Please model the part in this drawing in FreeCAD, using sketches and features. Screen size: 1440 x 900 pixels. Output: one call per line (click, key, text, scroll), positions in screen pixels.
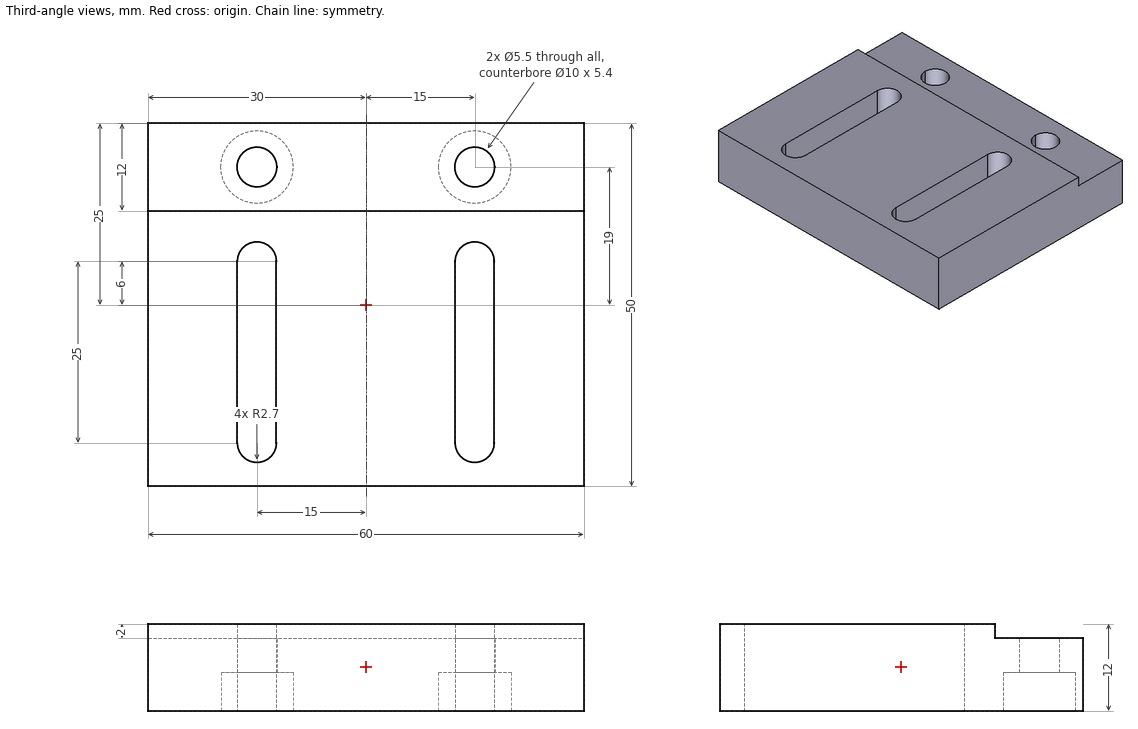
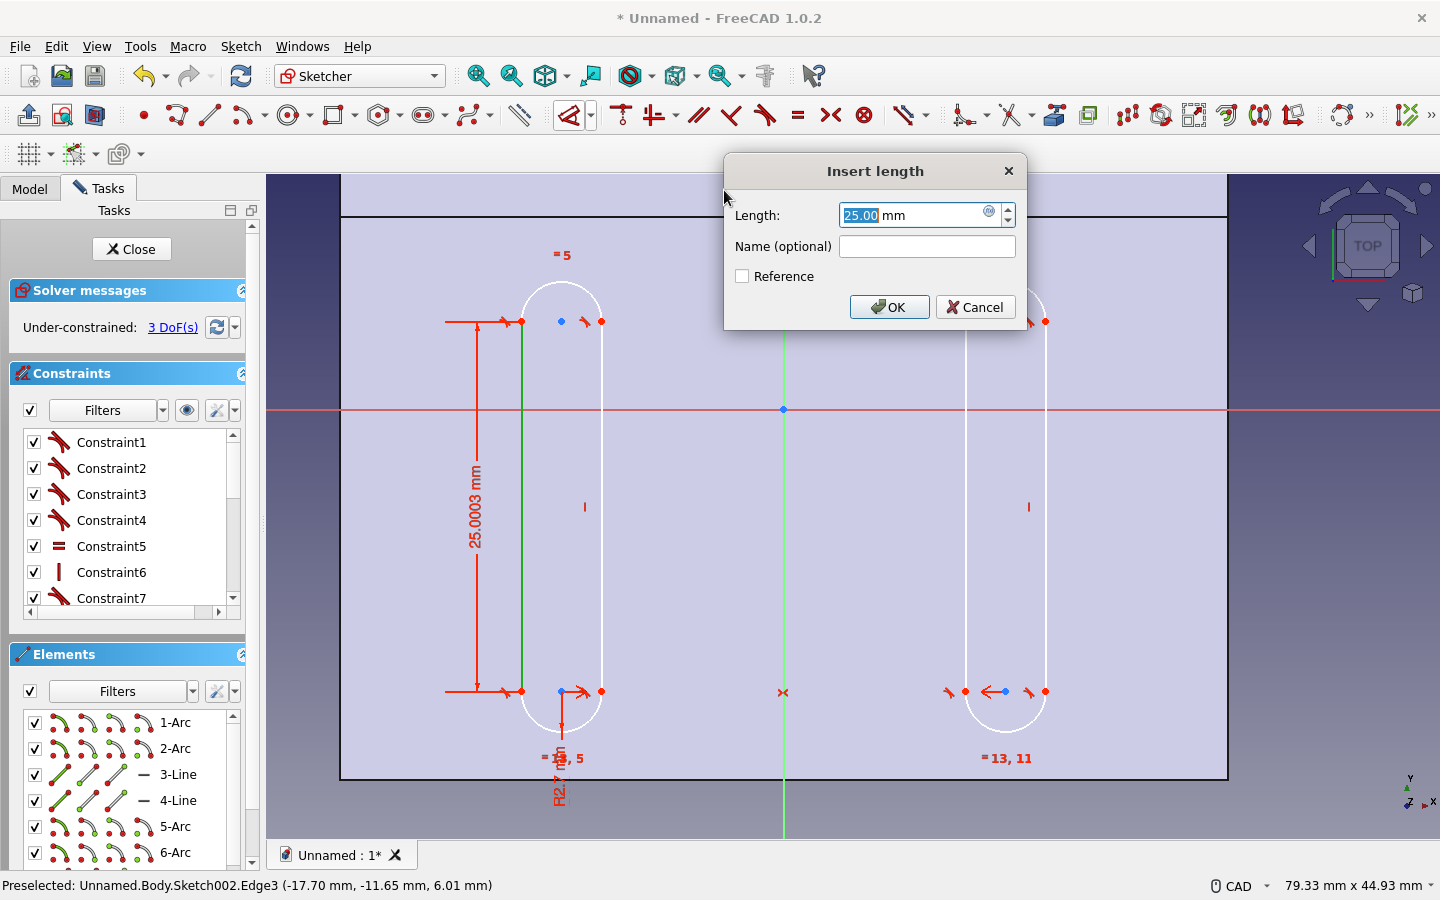
text(25)
key(Return)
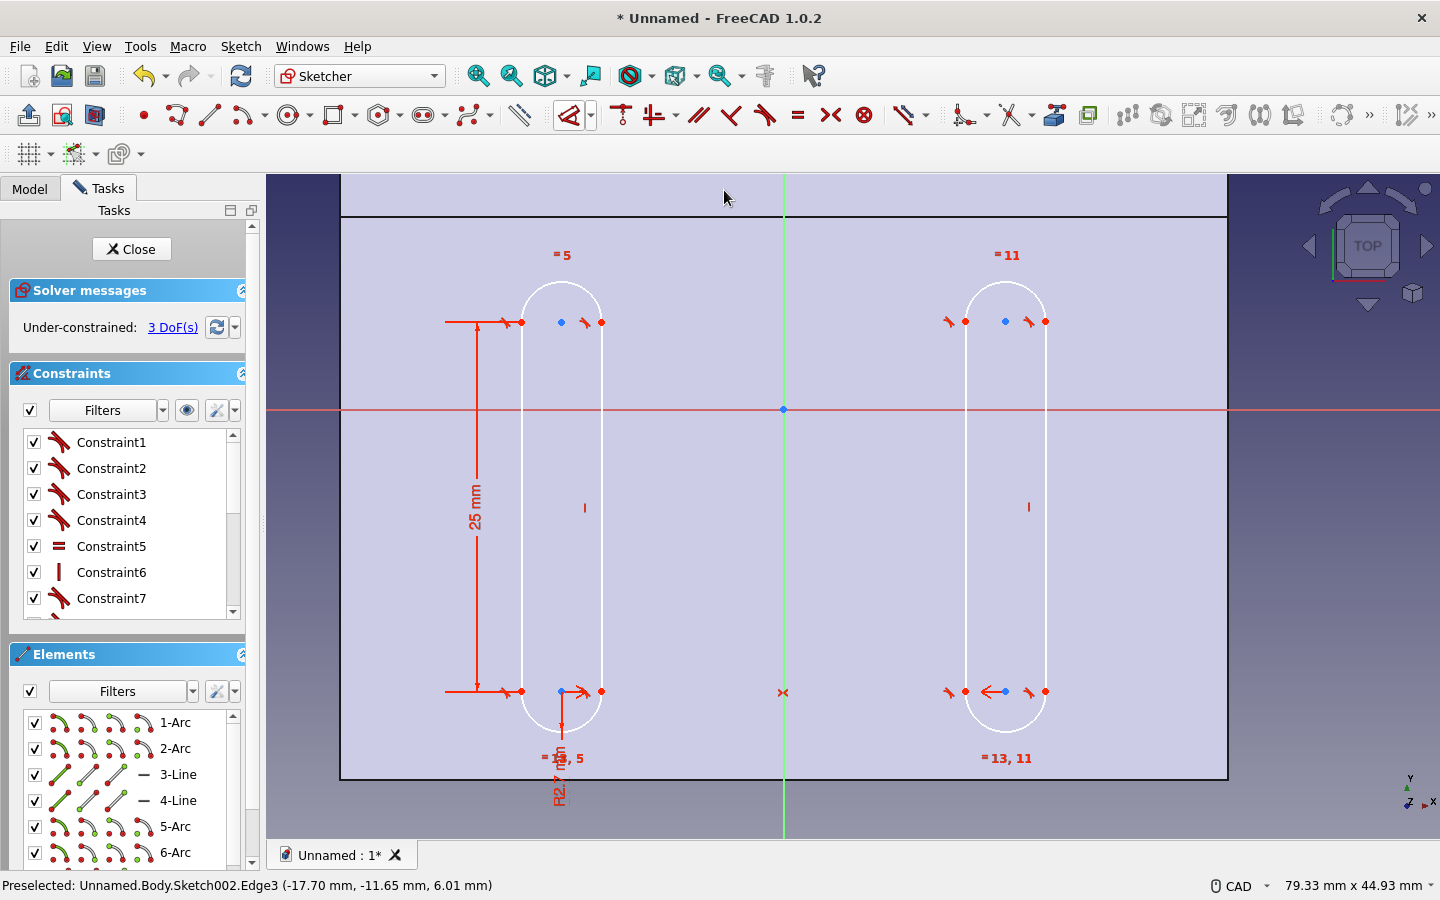
click(966, 581)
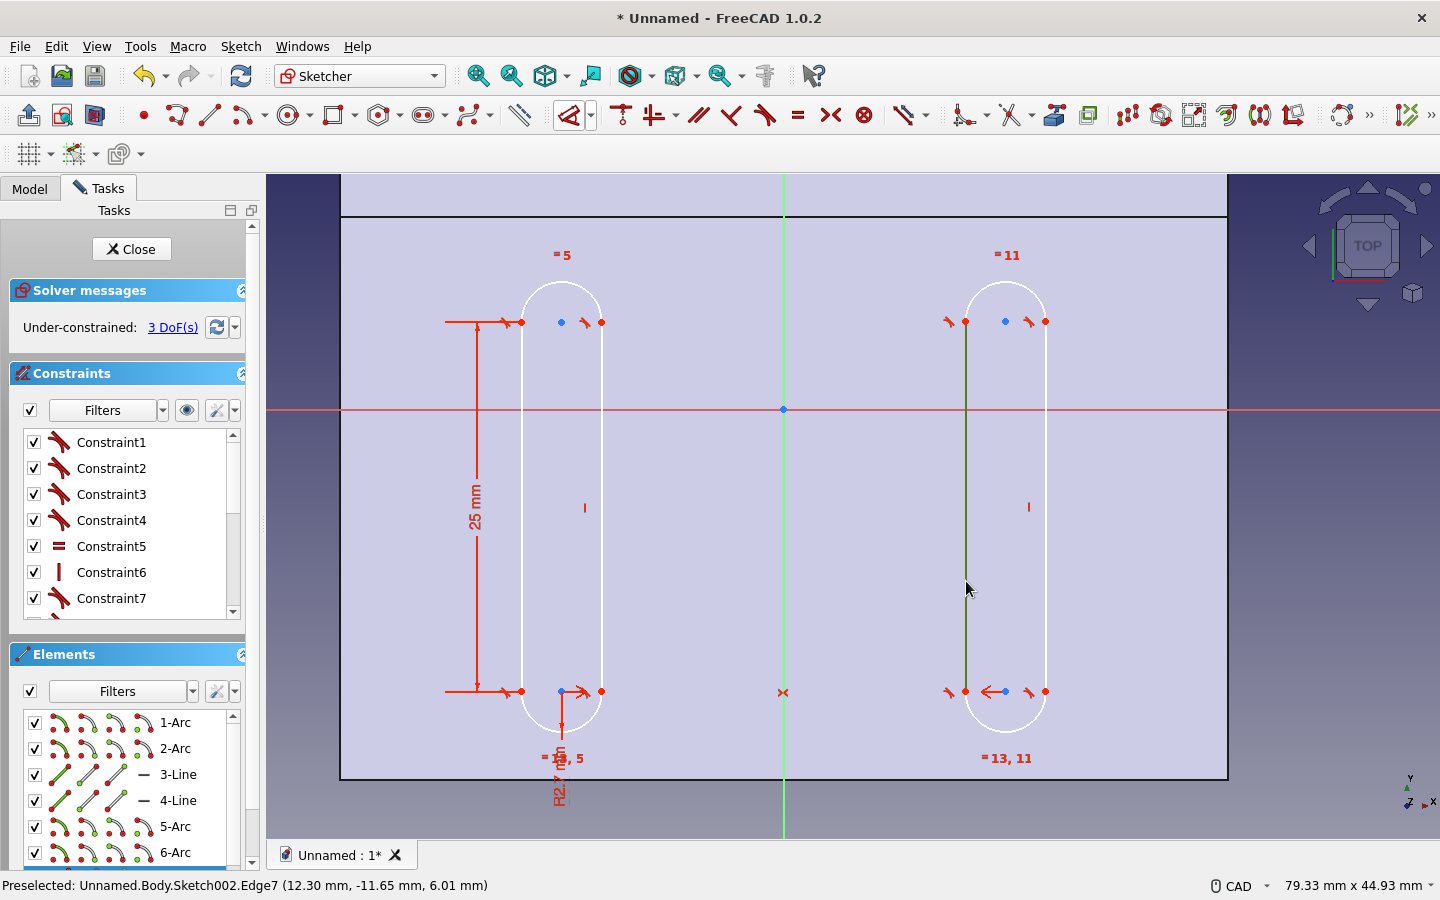
key(i)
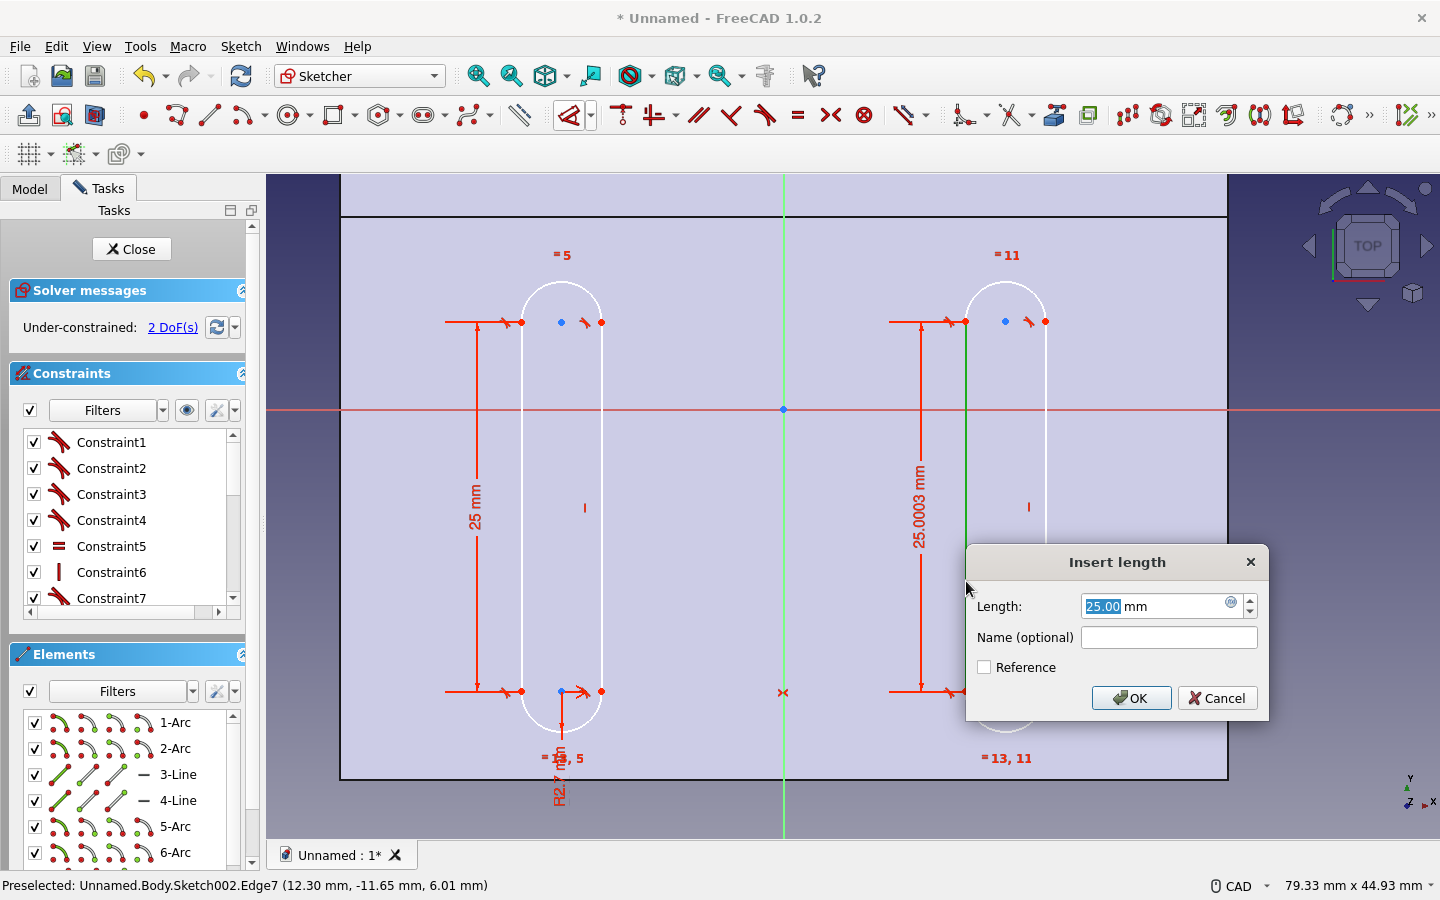
text(25)
key(Return)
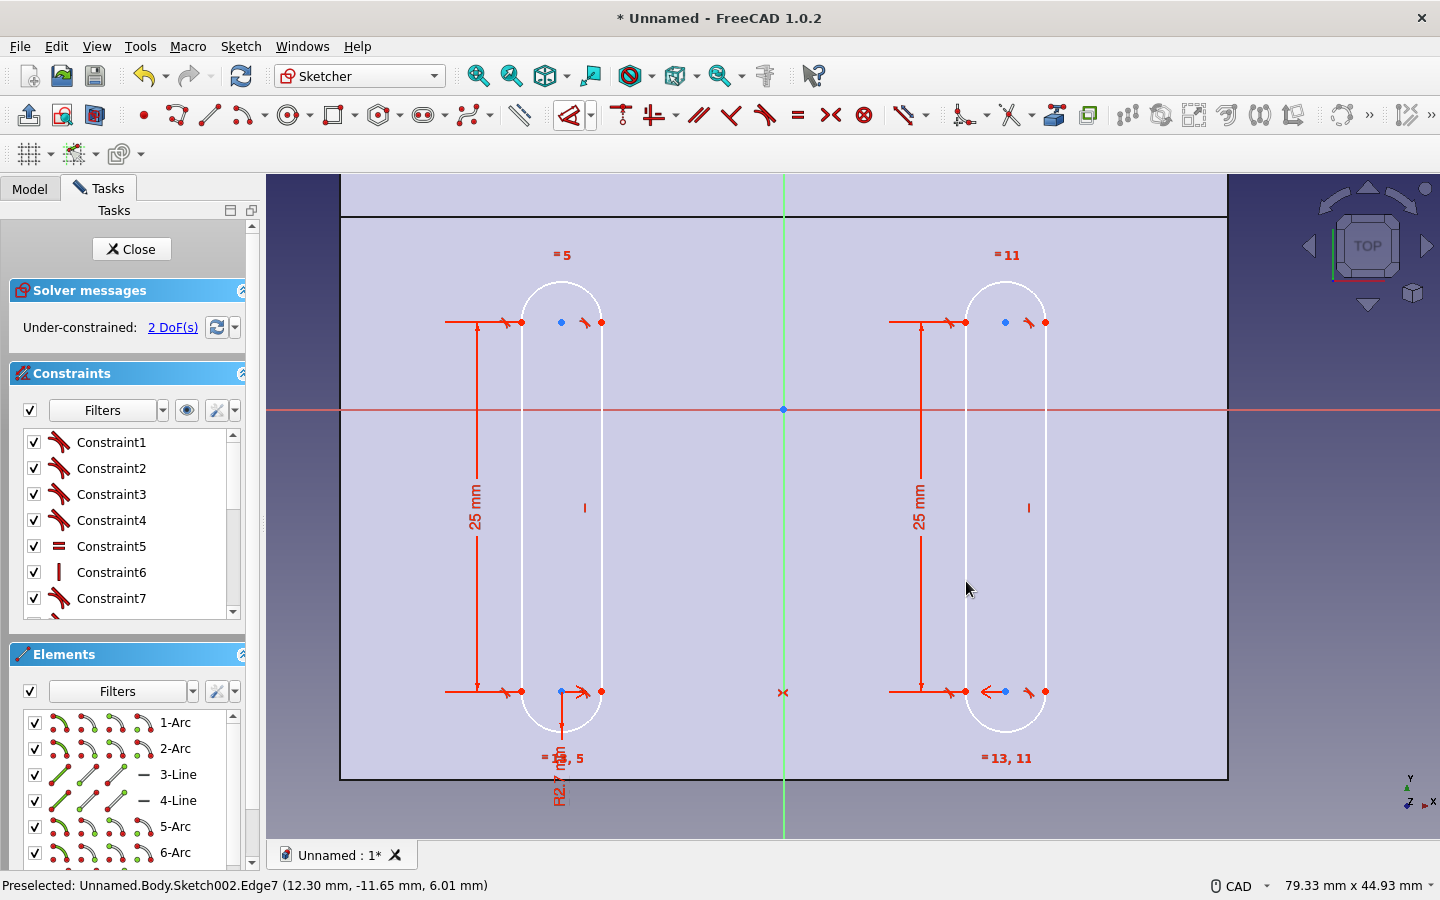
click(602, 322)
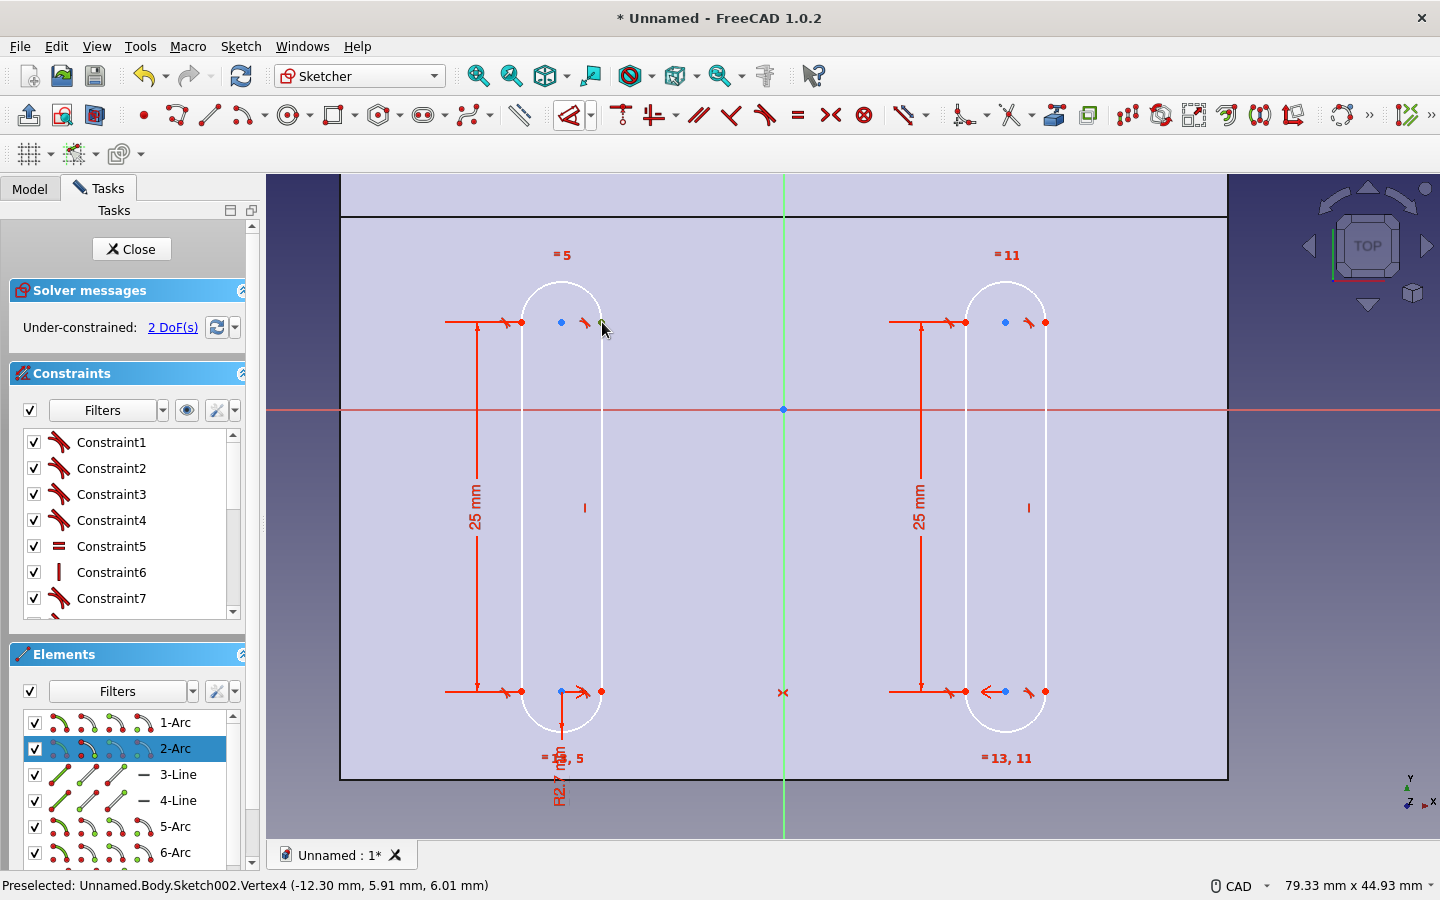
key(i)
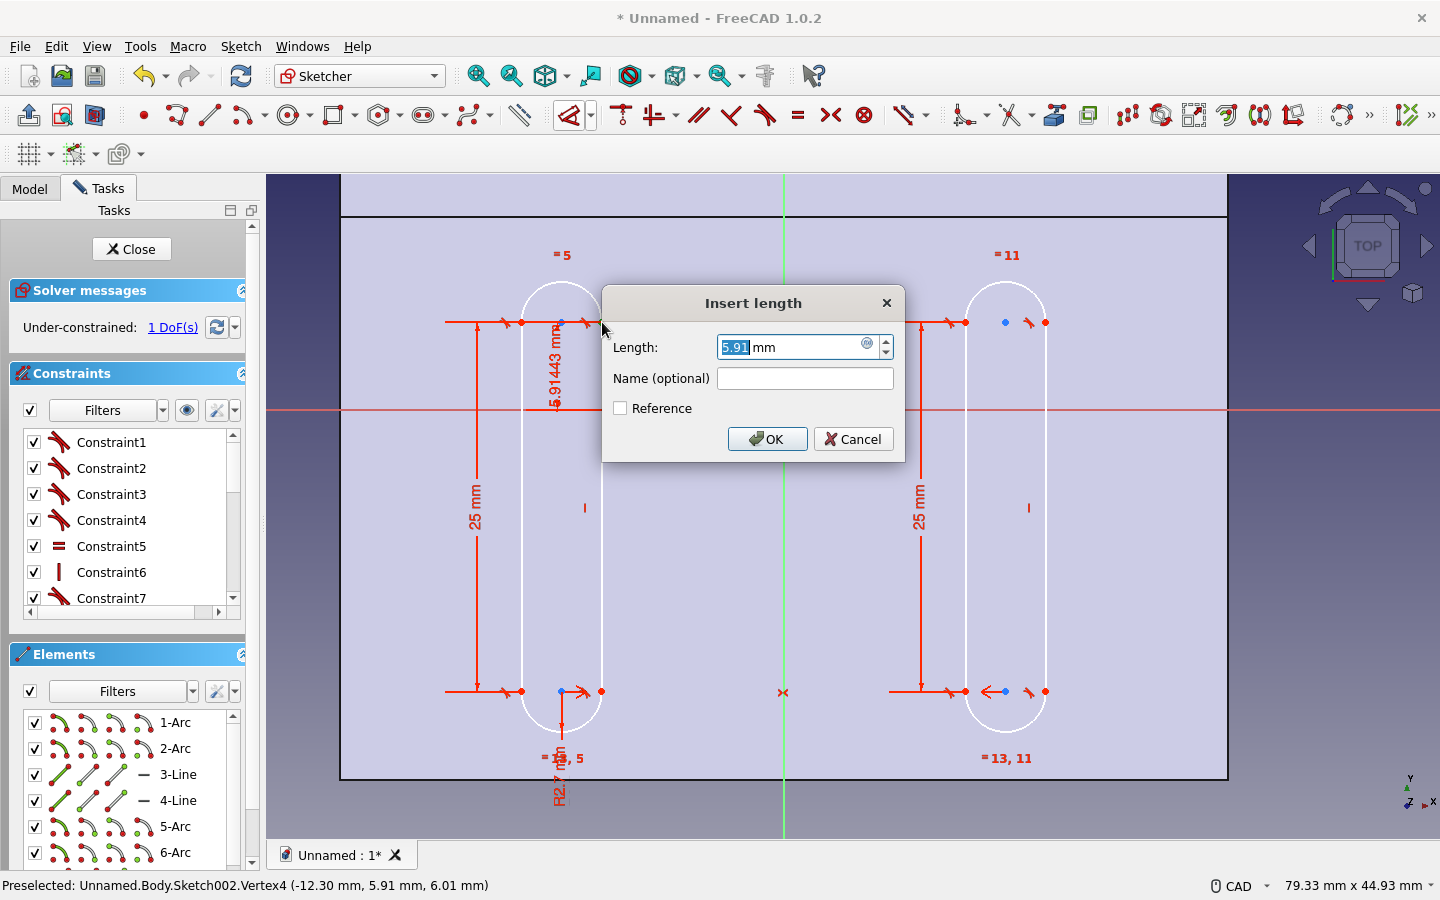
text(6)
key(Return)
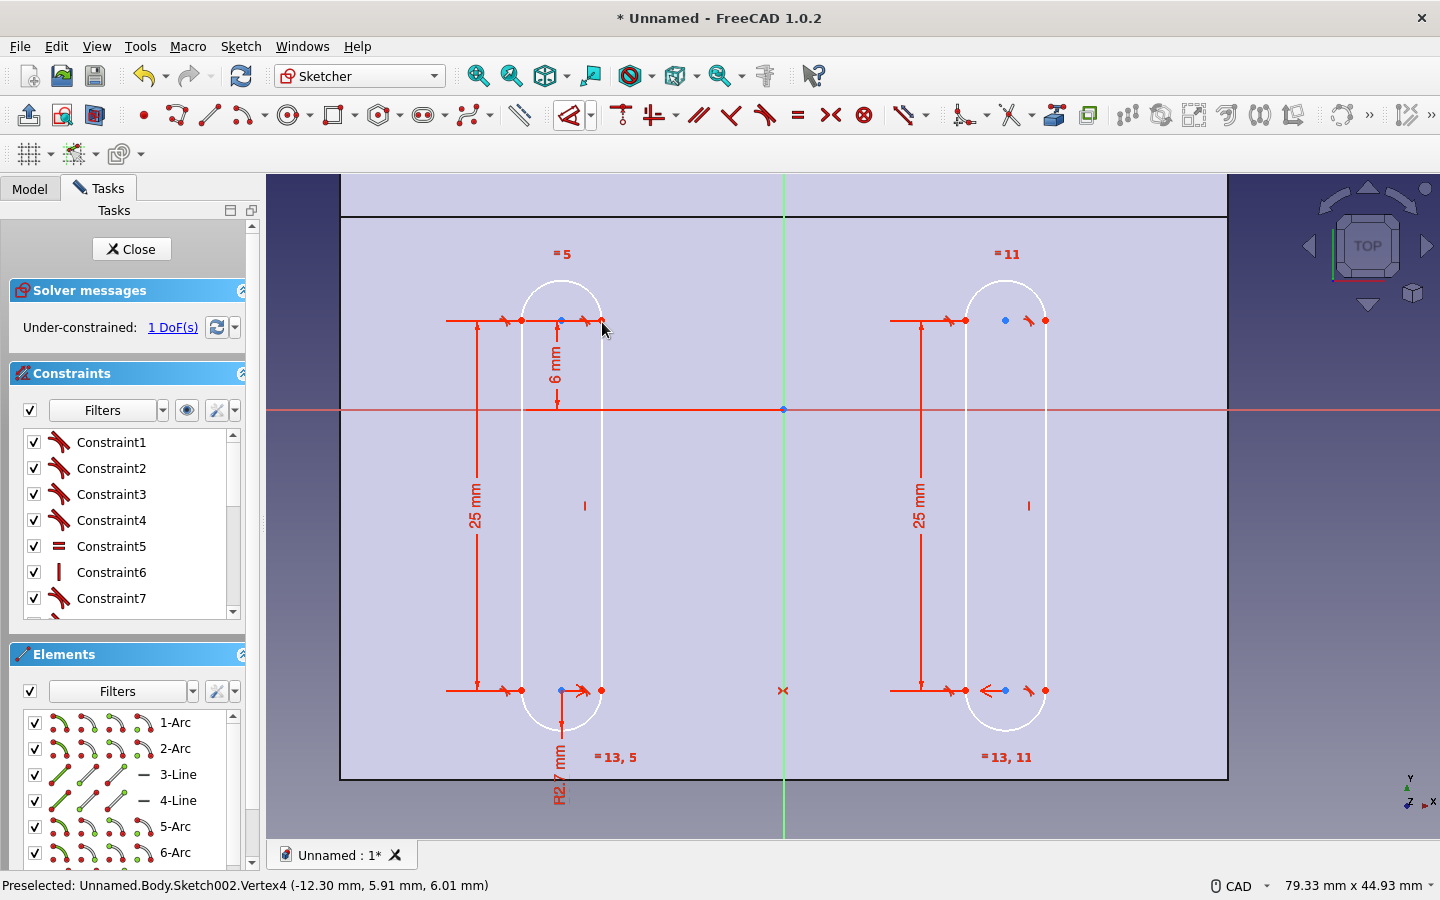
click(562, 691)